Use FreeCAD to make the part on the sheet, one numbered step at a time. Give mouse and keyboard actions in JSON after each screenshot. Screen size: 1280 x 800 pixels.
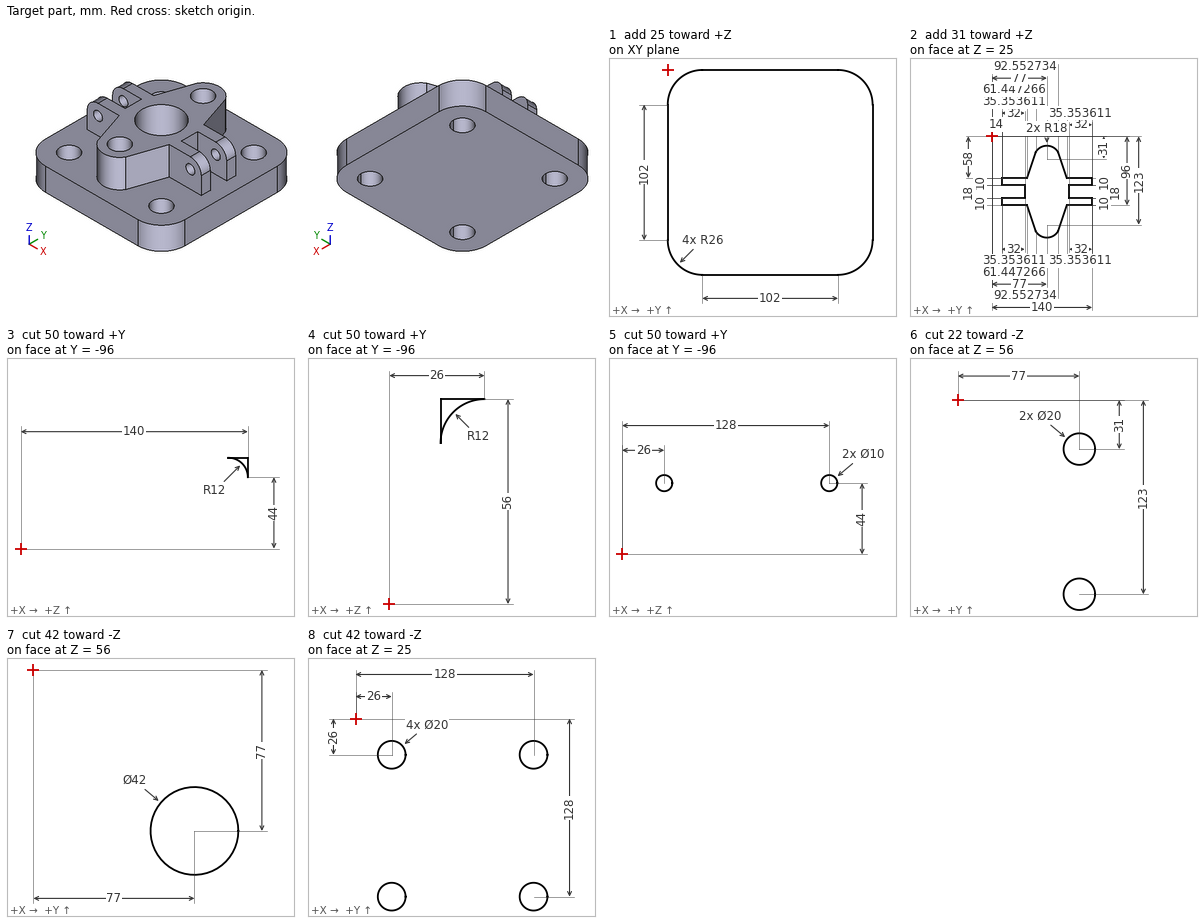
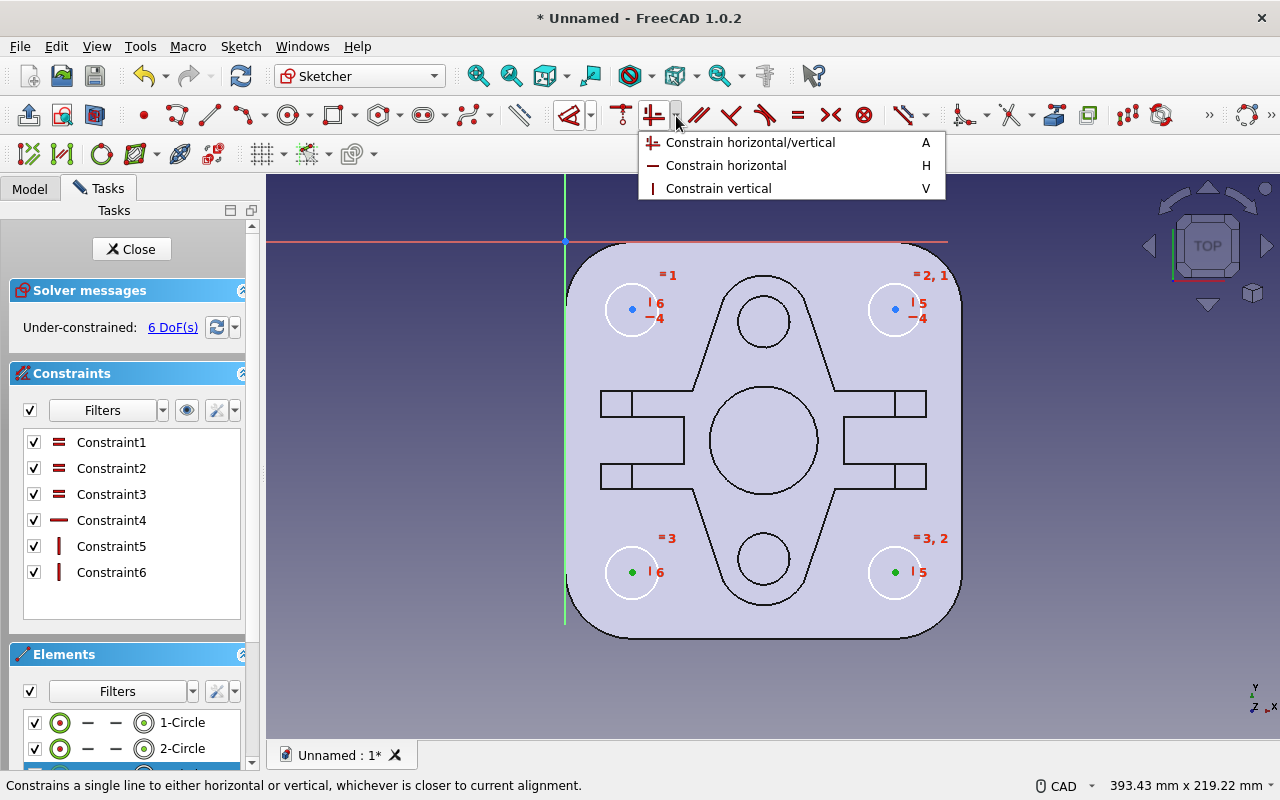
{"action": "left_click", "coordinate": [792, 166]}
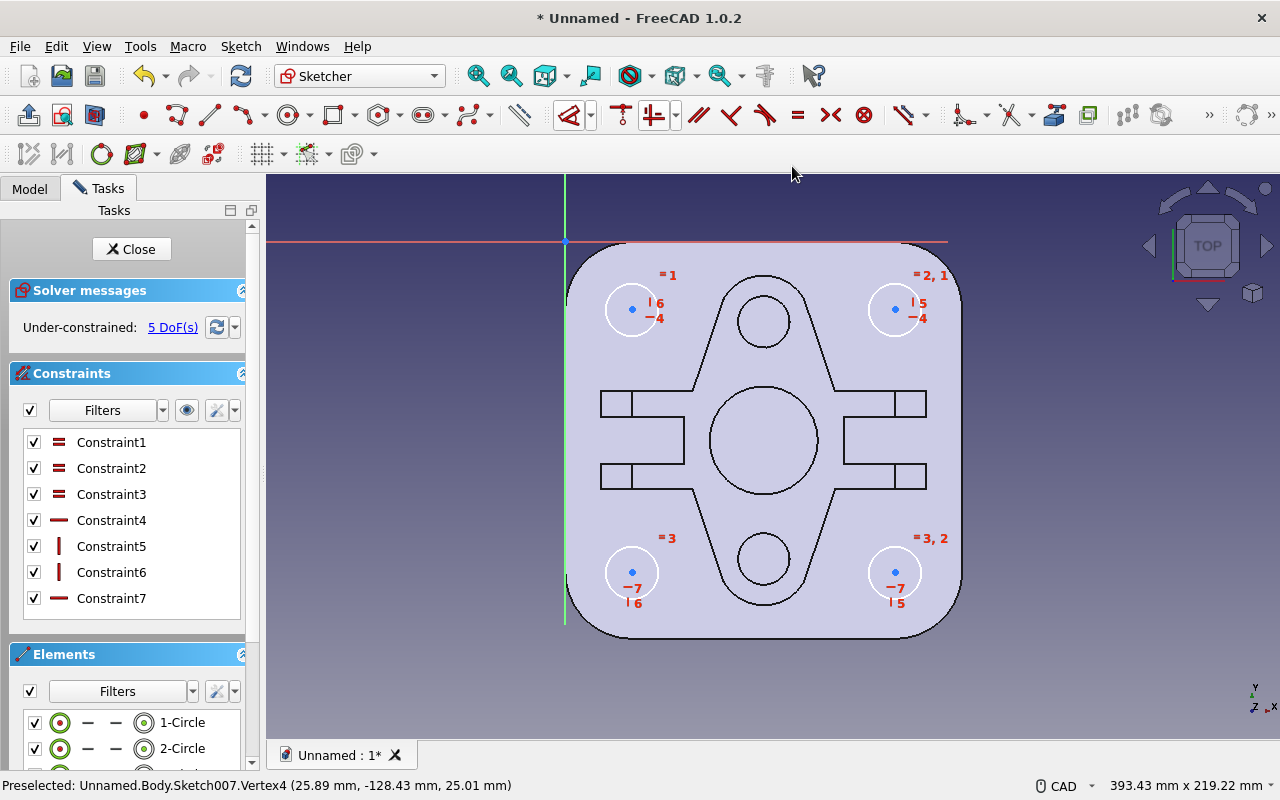
{"action": "left_click", "coordinate": [650, 291]}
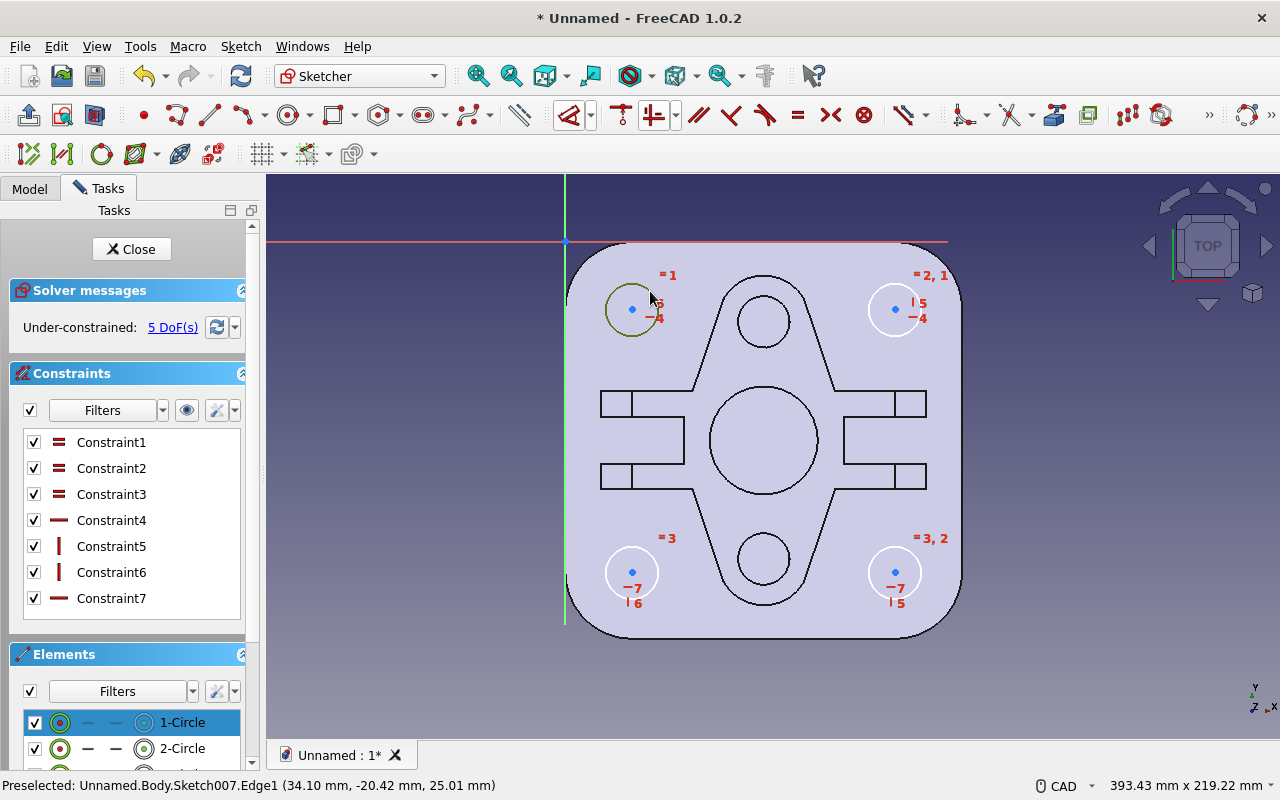
{"action": "left_click", "coordinate": [590, 116]}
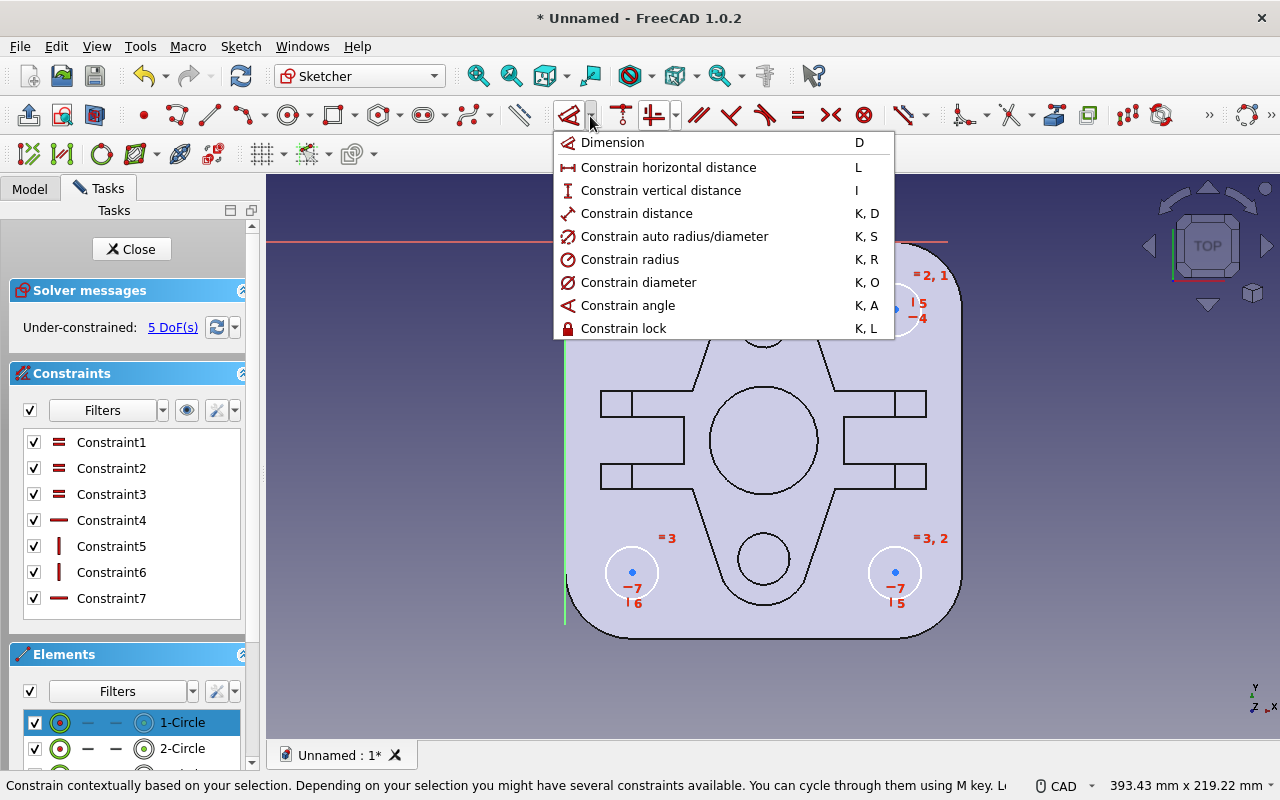
{"action": "left_click", "coordinate": [724, 282]}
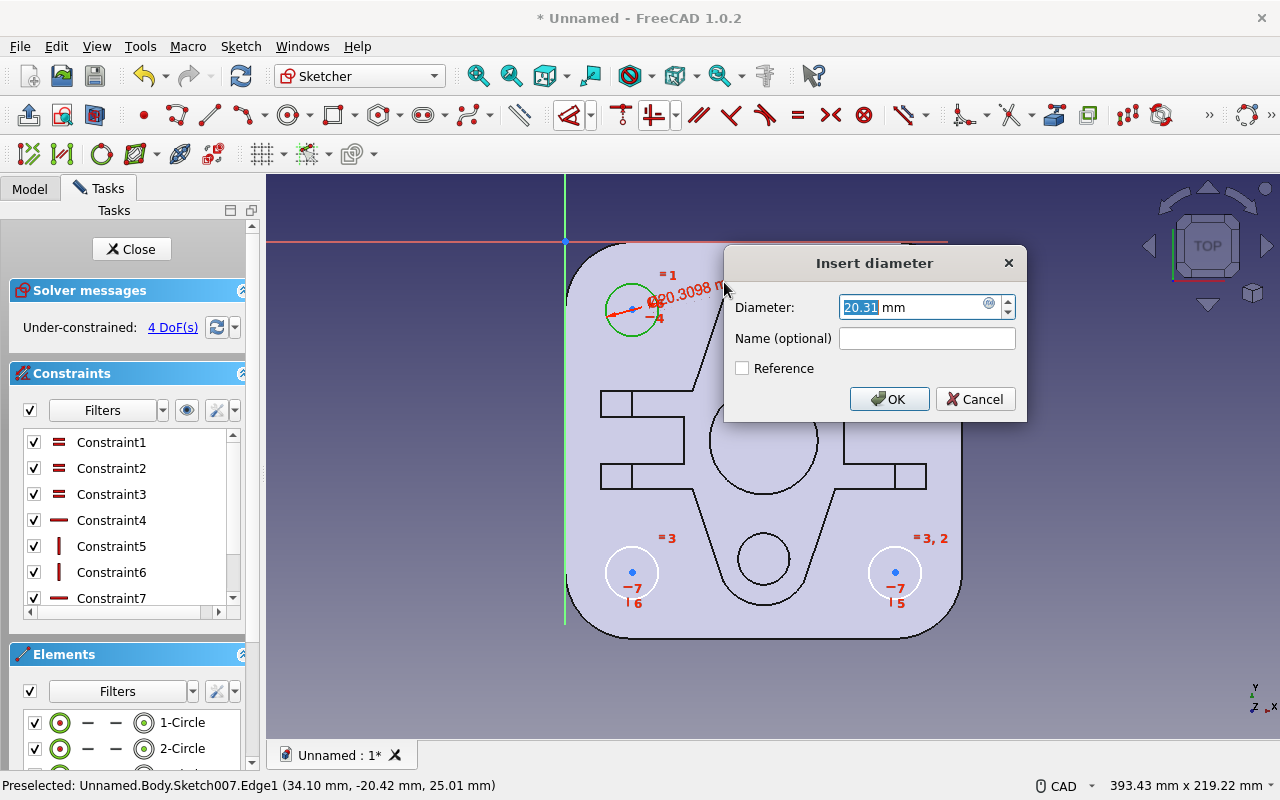
{"action": "type", "text": "20"}
{"action": "key", "text": "Return"}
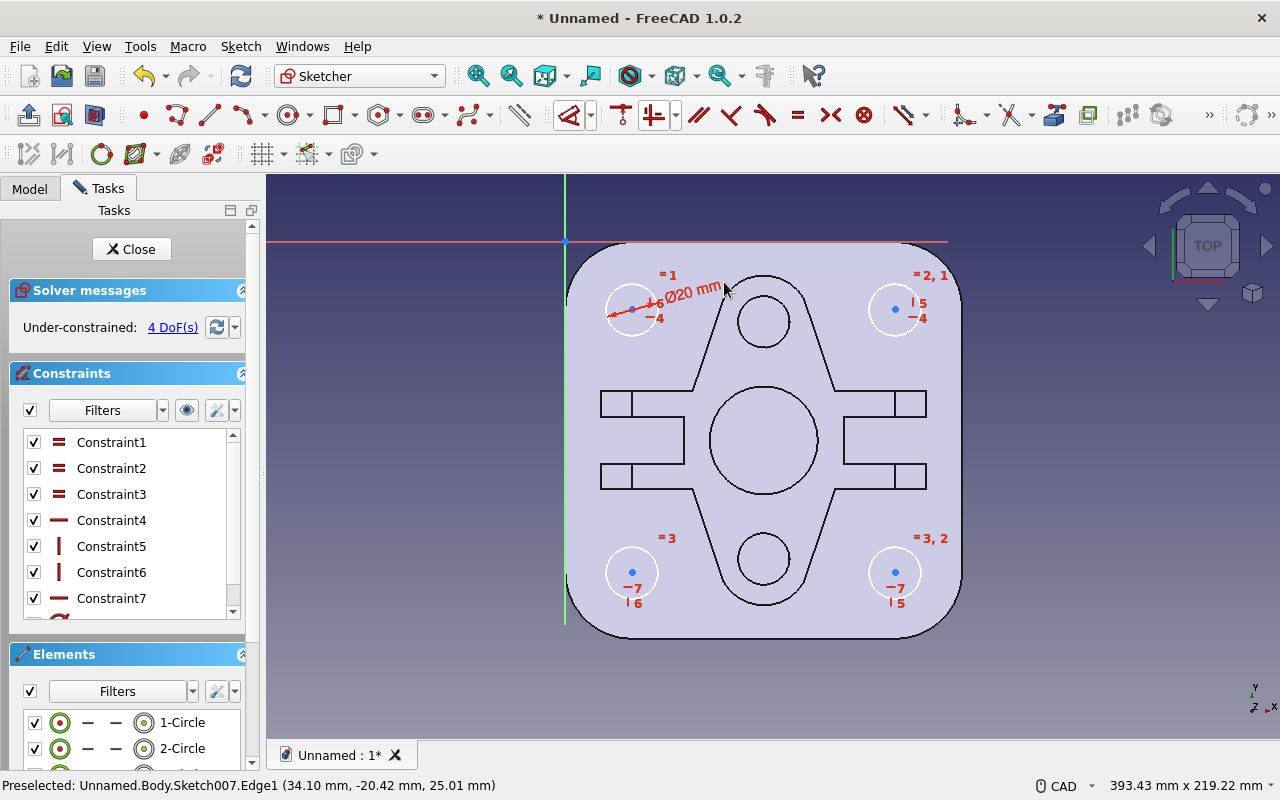
{"action": "left_click", "coordinate": [632, 310]}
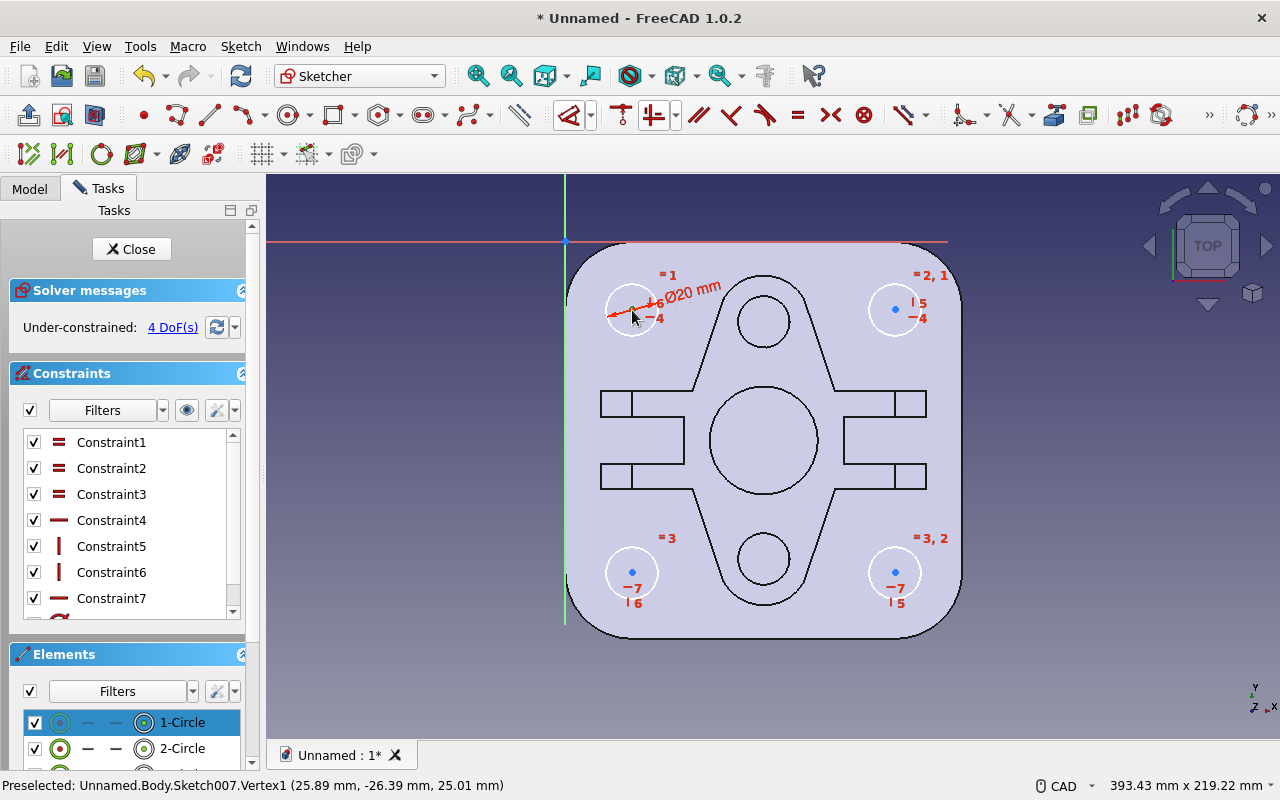
{"action": "key", "text": "l"}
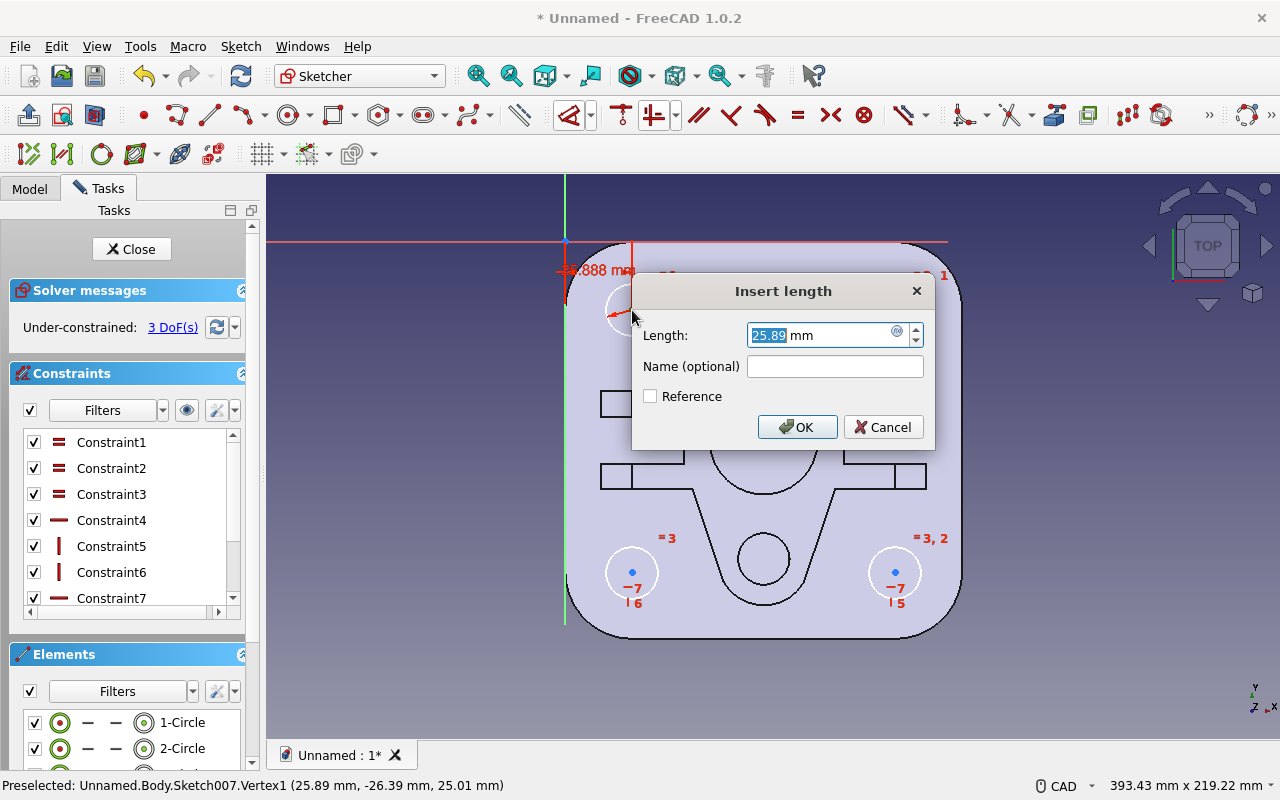
{"action": "type", "text": "26"}
{"action": "key", "text": "Return"}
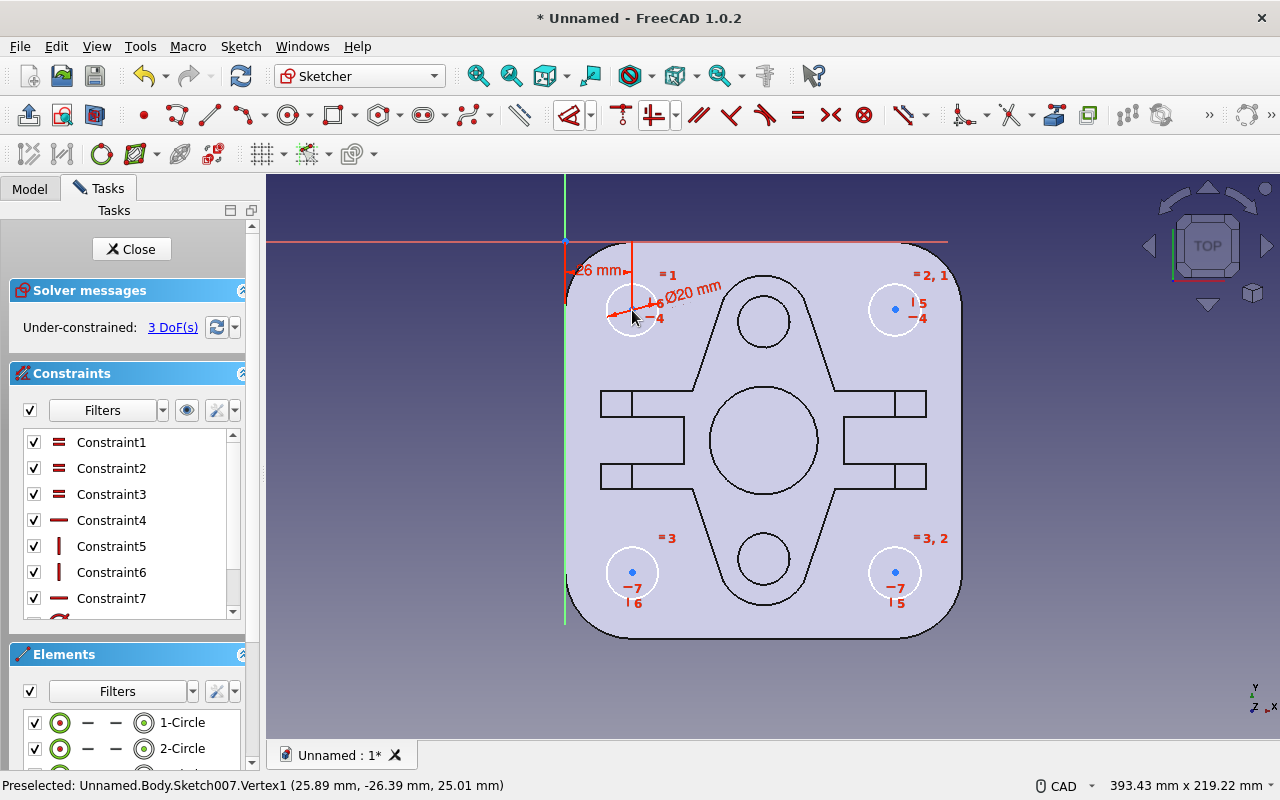
{"action": "left_click", "coordinate": [632, 310]}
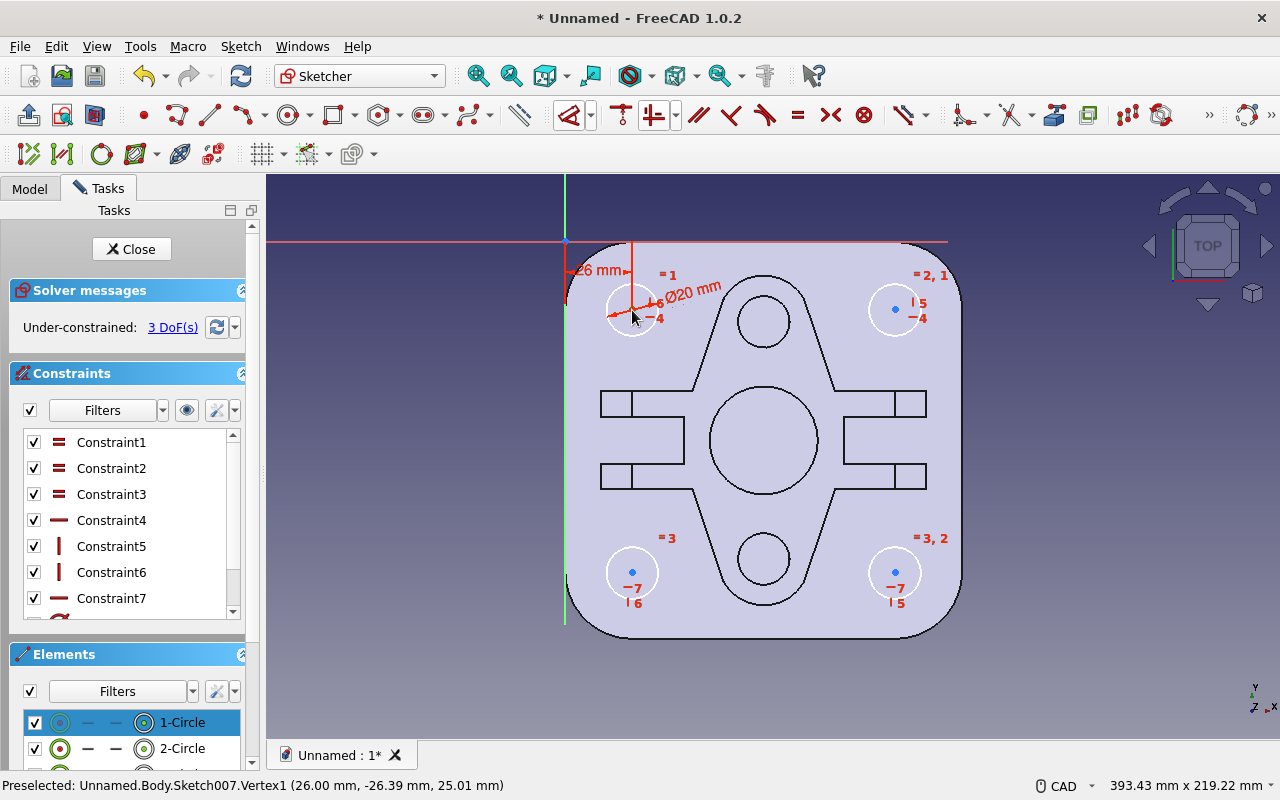
{"action": "left_click", "coordinate": [590, 116]}